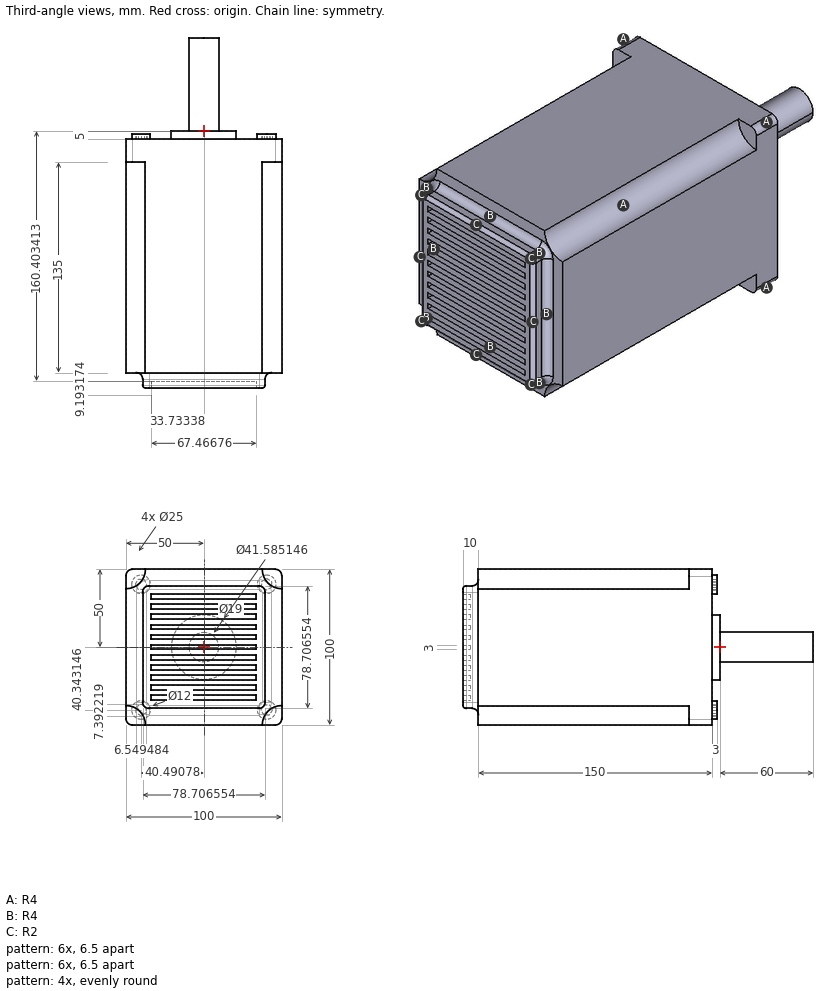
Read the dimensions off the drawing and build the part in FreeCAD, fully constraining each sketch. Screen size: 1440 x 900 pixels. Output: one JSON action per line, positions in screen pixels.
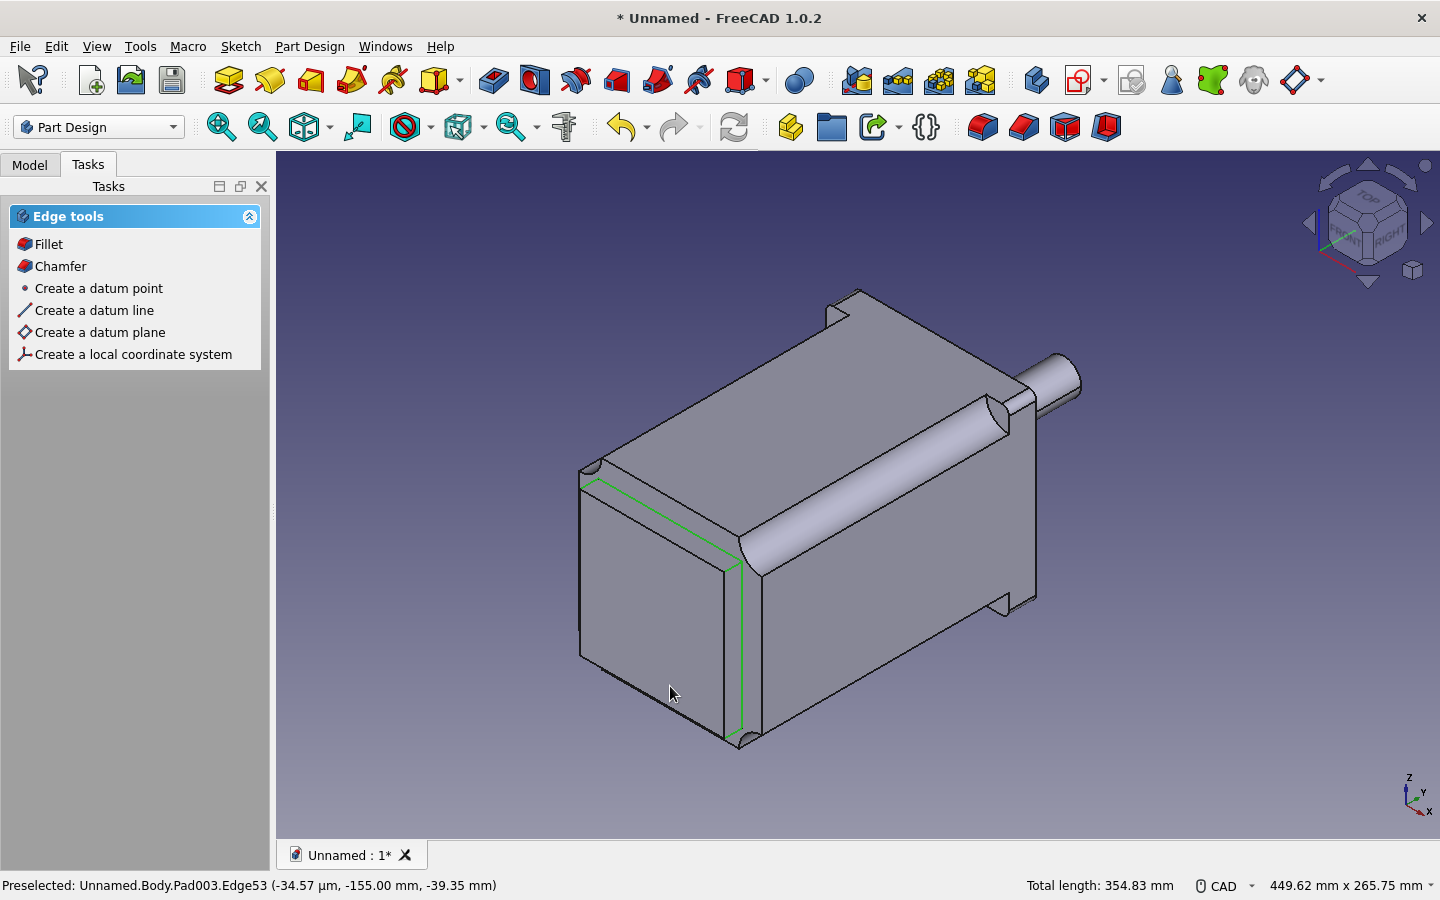
{"action": "left_click", "coordinate": [983, 128]}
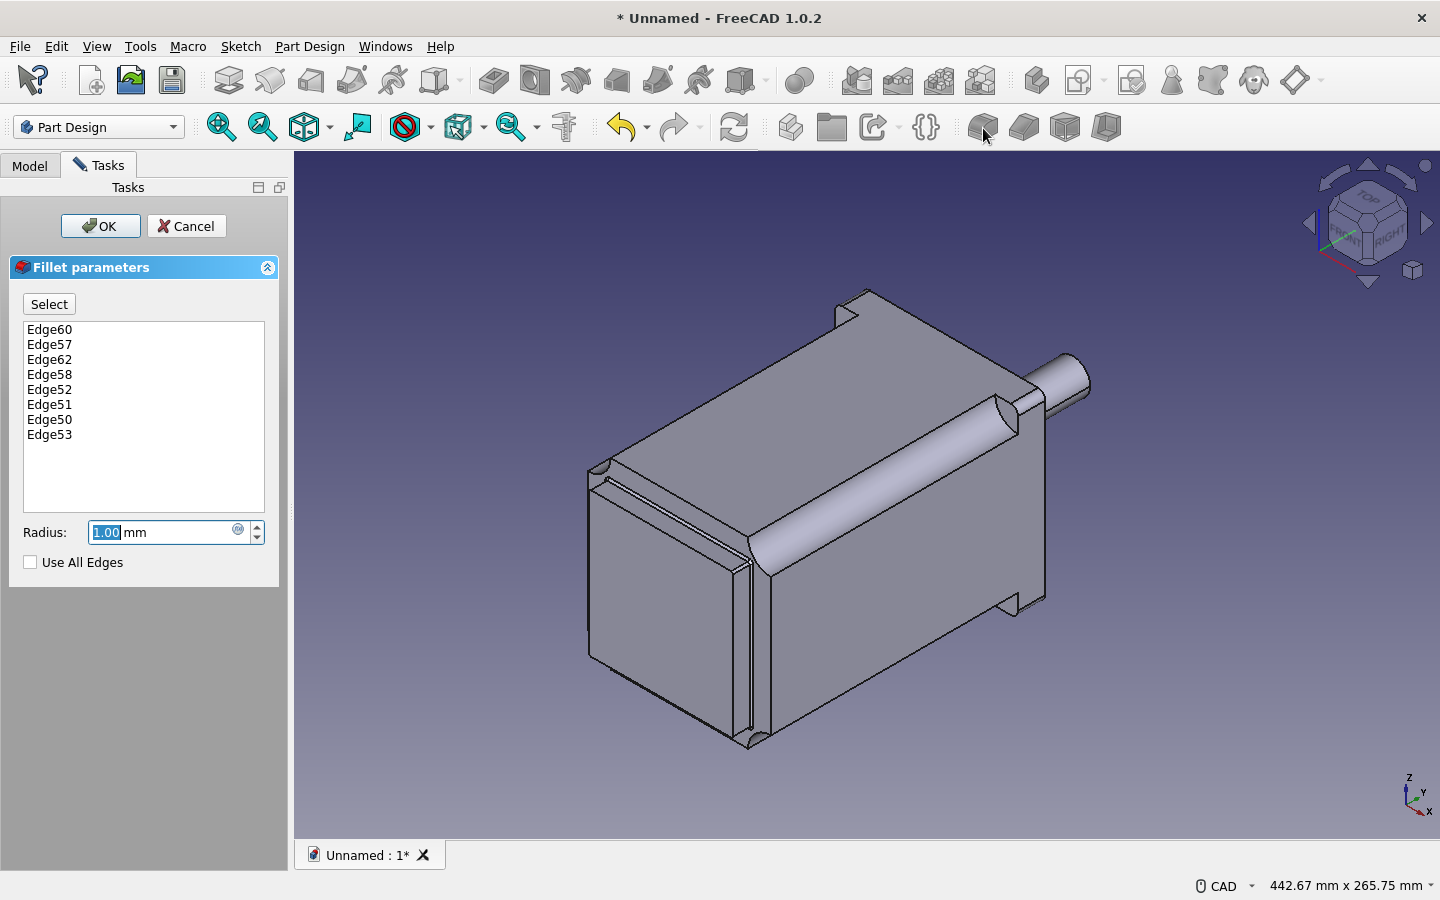
{"action": "type", "text": "4"}
{"action": "key", "text": "Tab"}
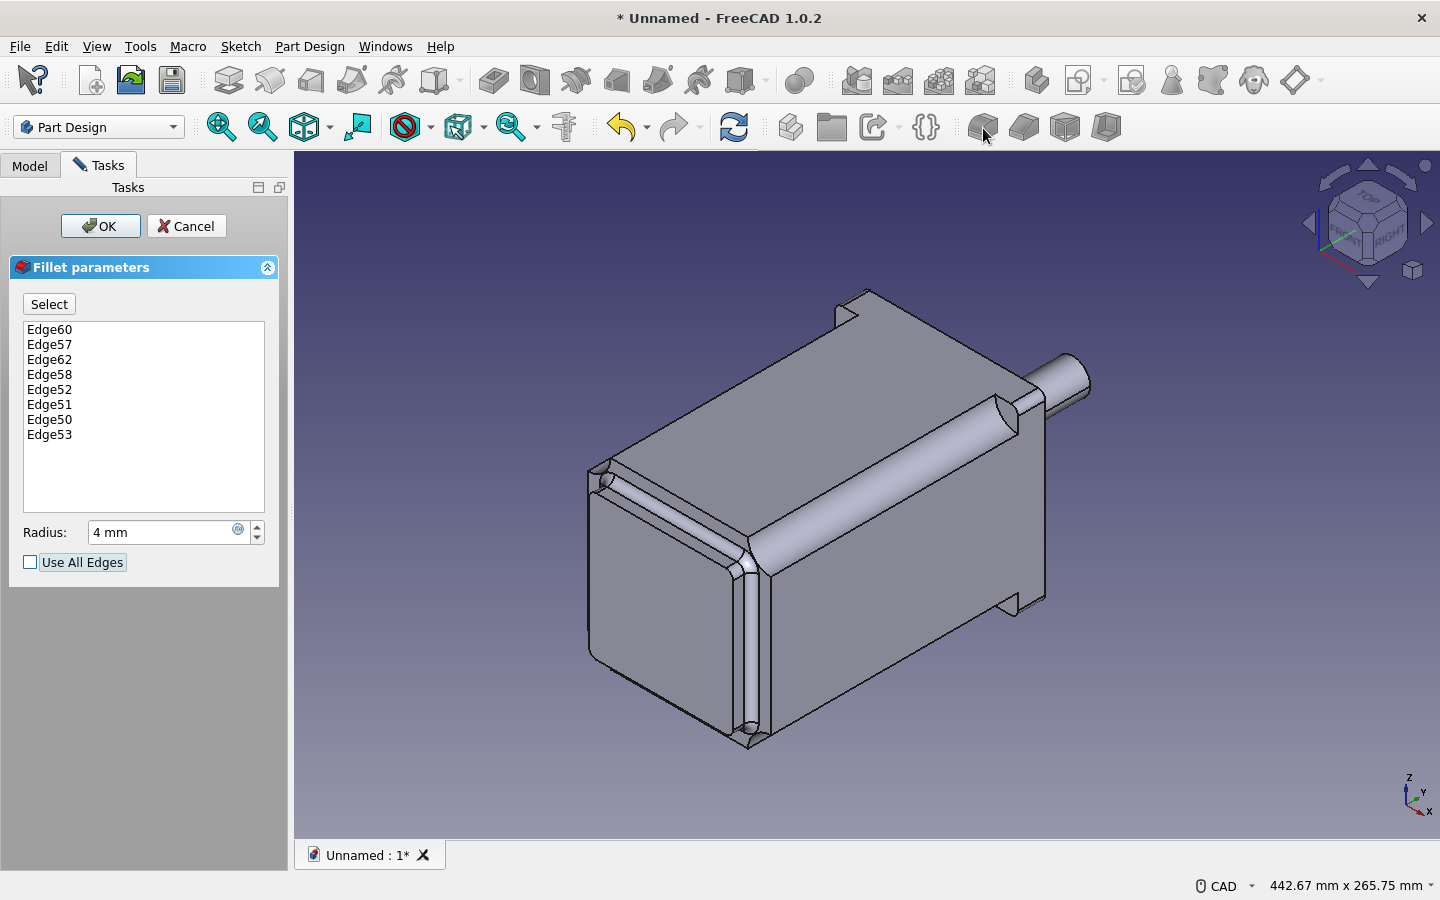
{"action": "left_click", "coordinate": [101, 226]}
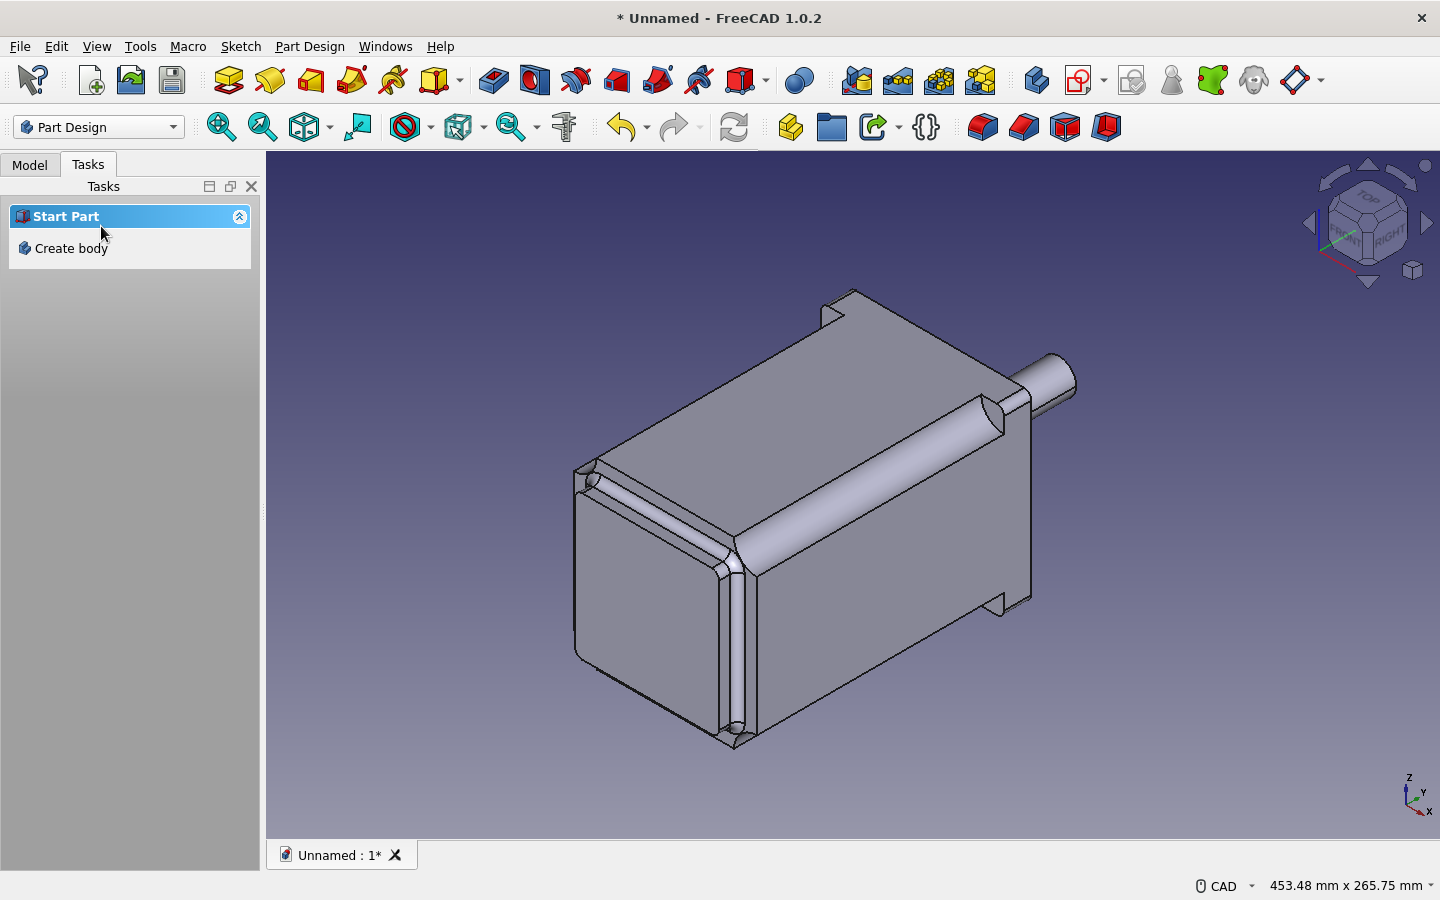
{"action": "left_click", "coordinate": [647, 613]}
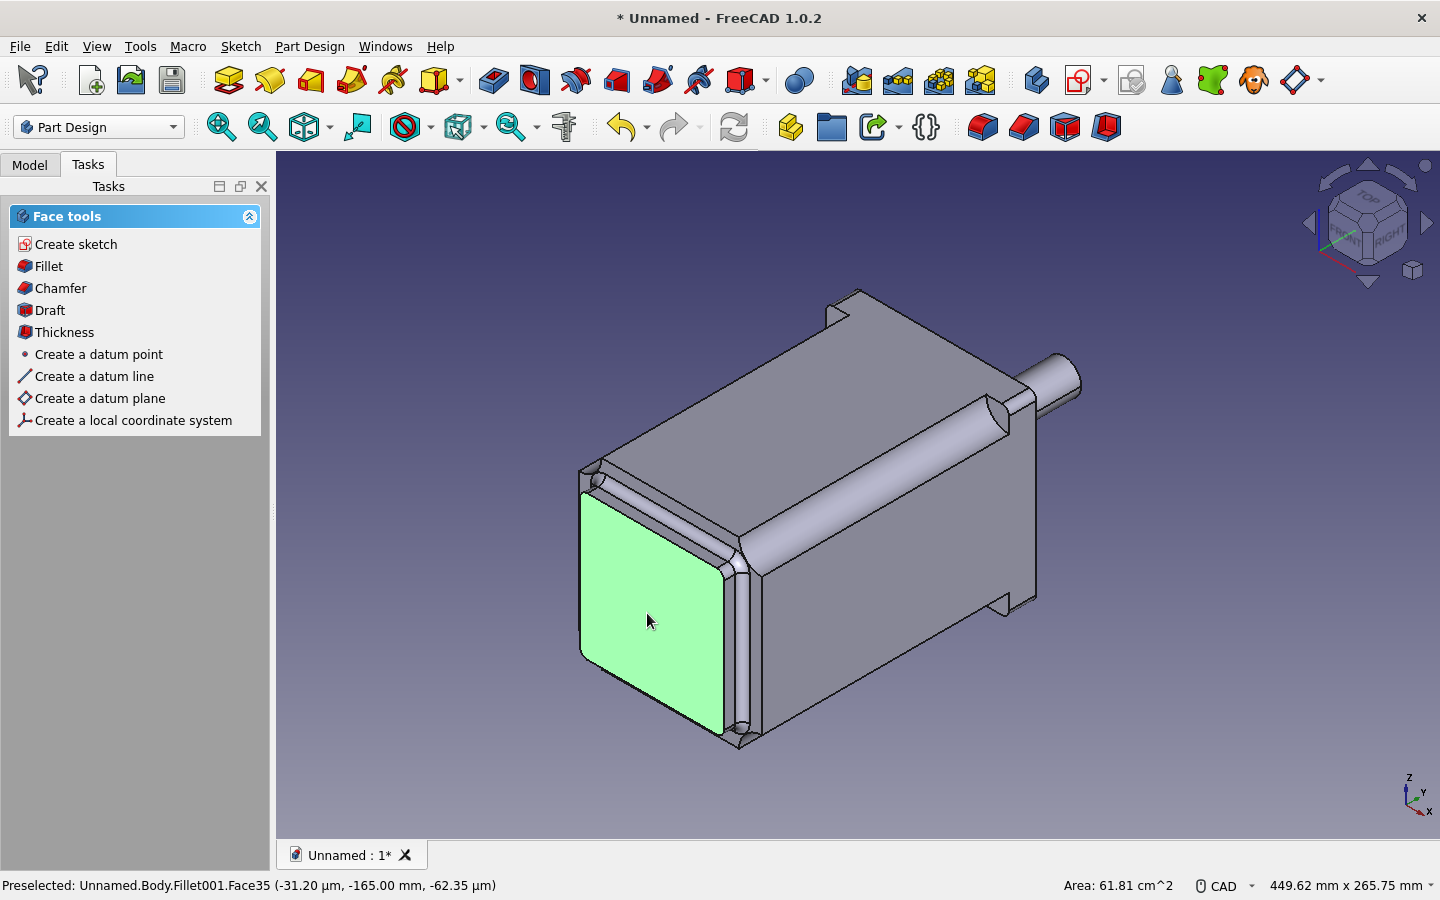
{"action": "left_click", "coordinate": [983, 128]}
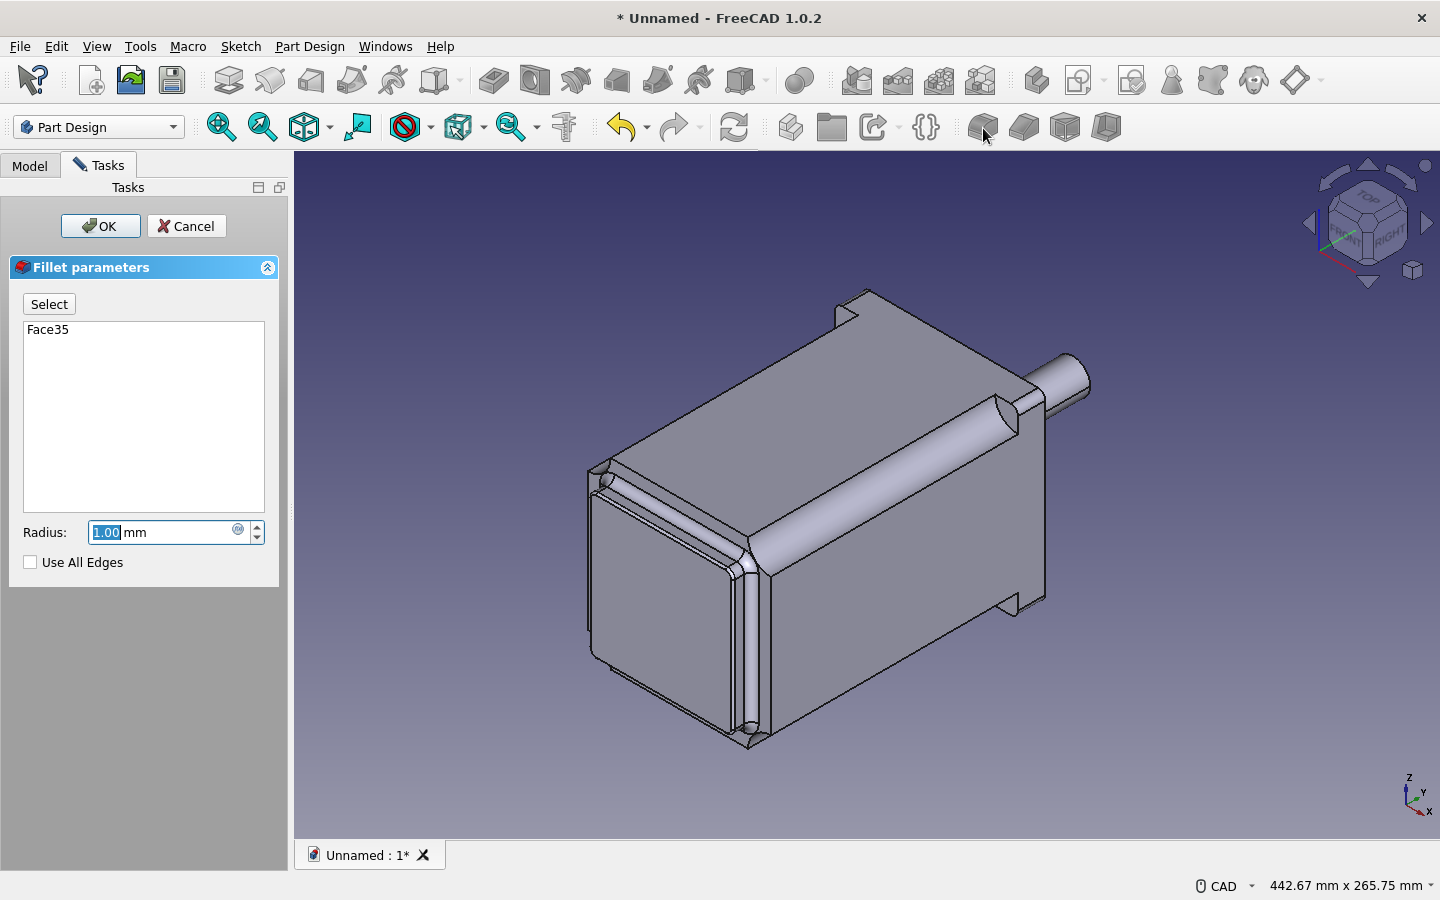
{"action": "type", "text": "2"}
{"action": "key", "text": "Tab"}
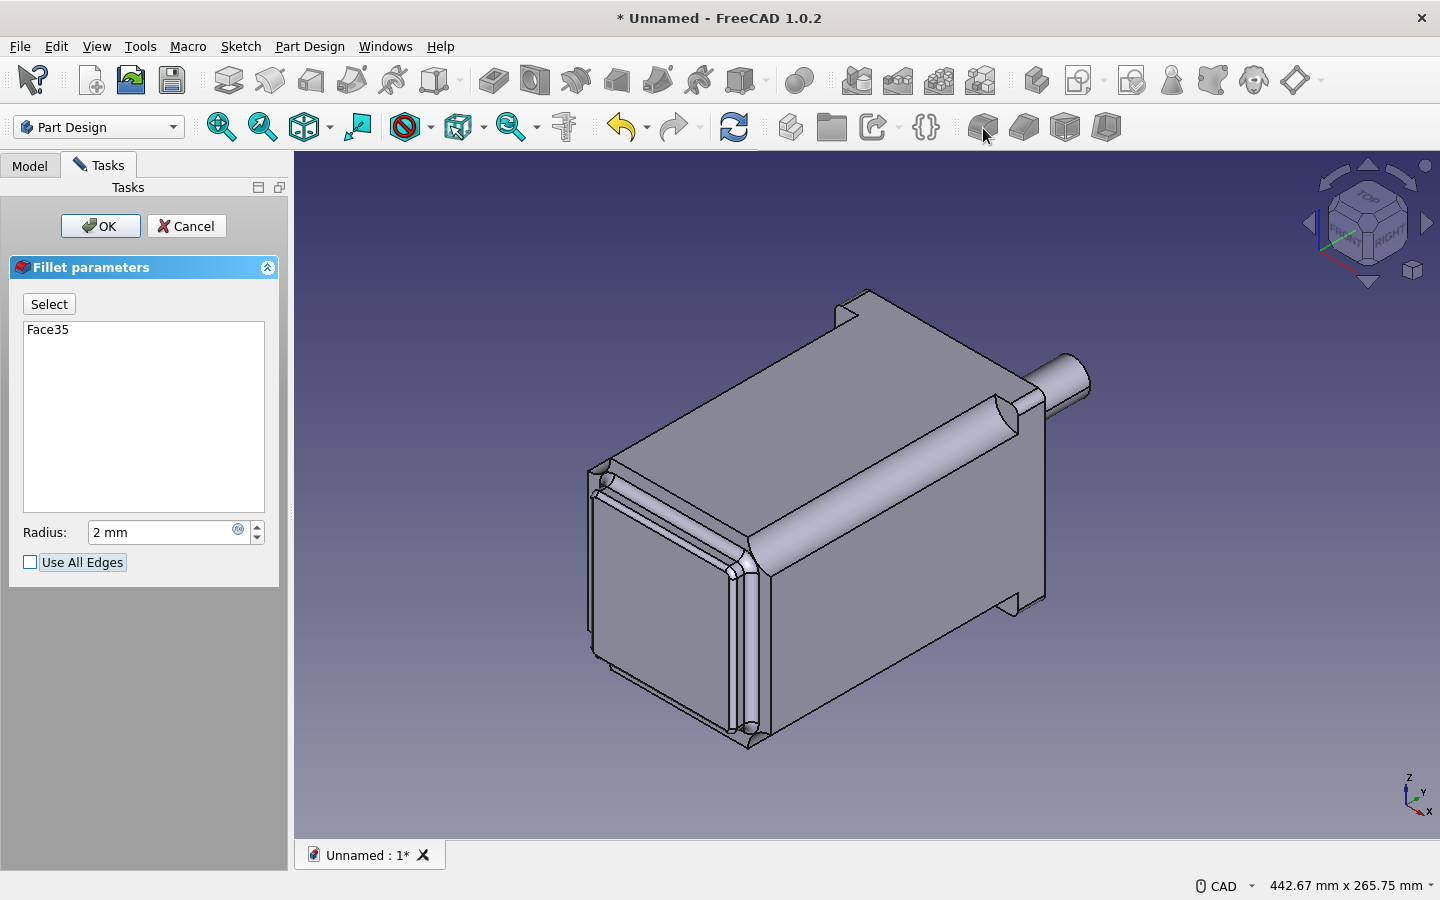
{"action": "left_click", "coordinate": [101, 226]}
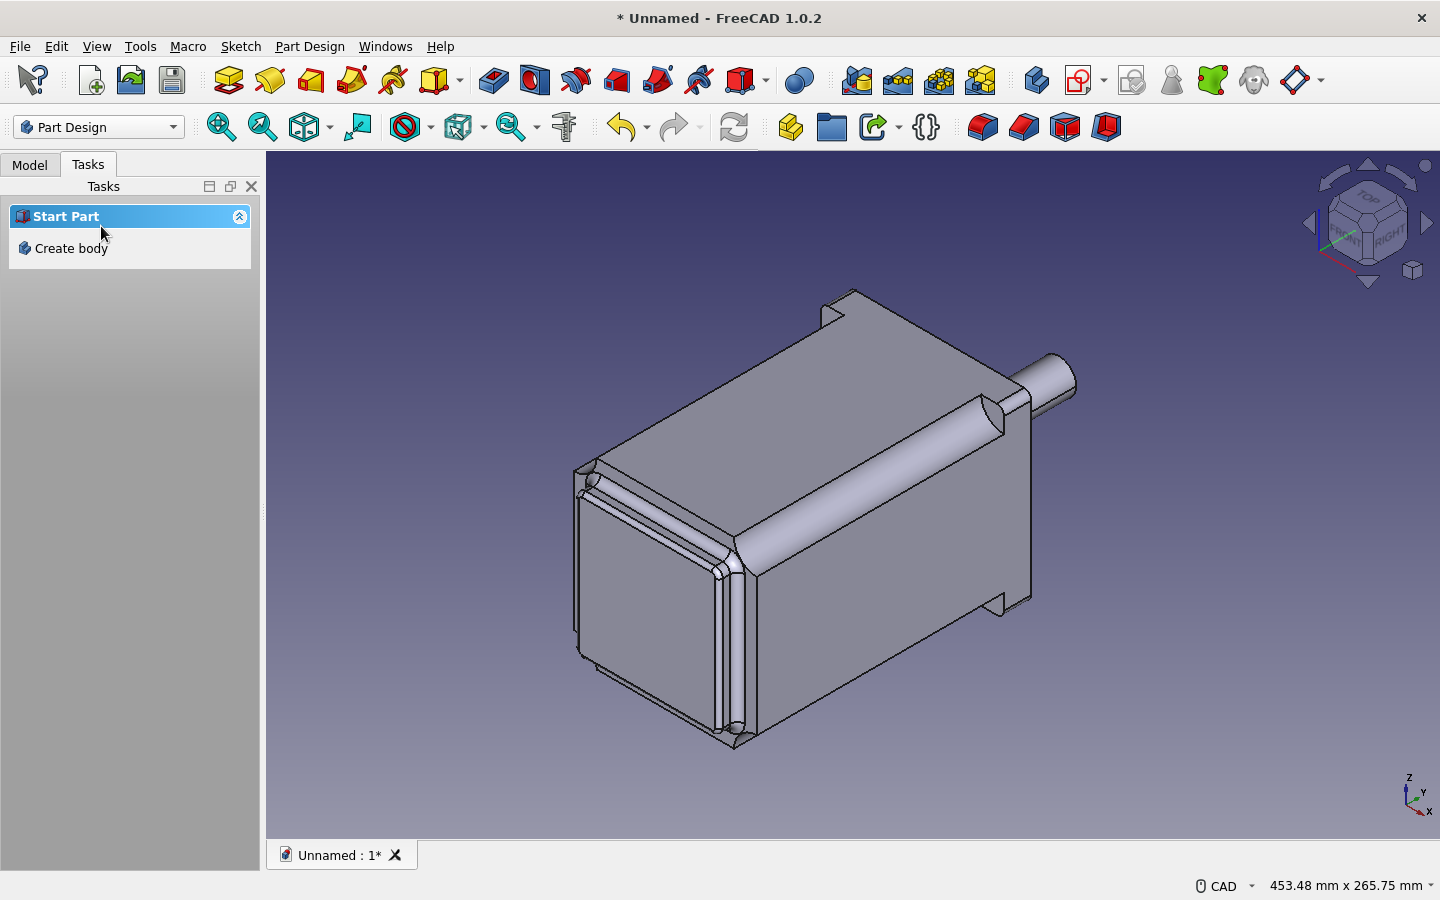
{"action": "left_click", "coordinate": [1078, 80]}